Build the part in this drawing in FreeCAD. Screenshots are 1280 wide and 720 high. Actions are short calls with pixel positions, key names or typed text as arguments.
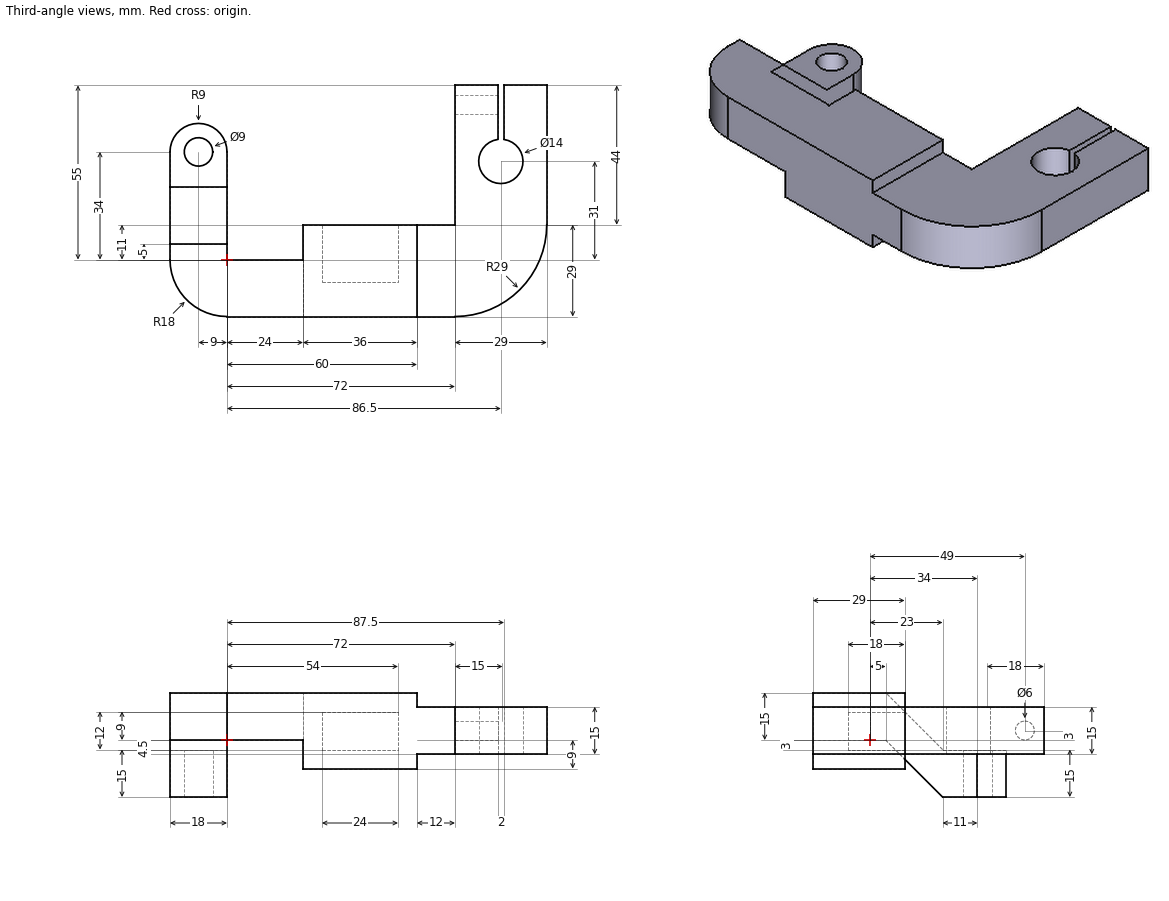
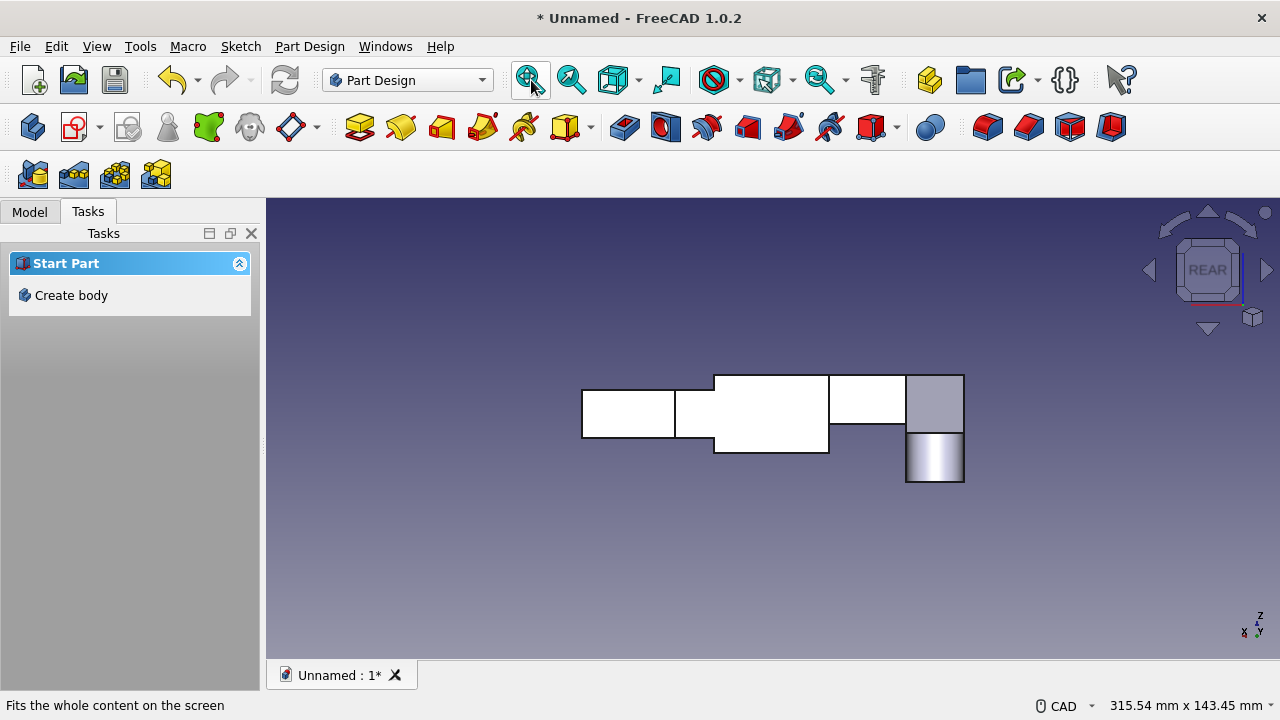
click(615, 413)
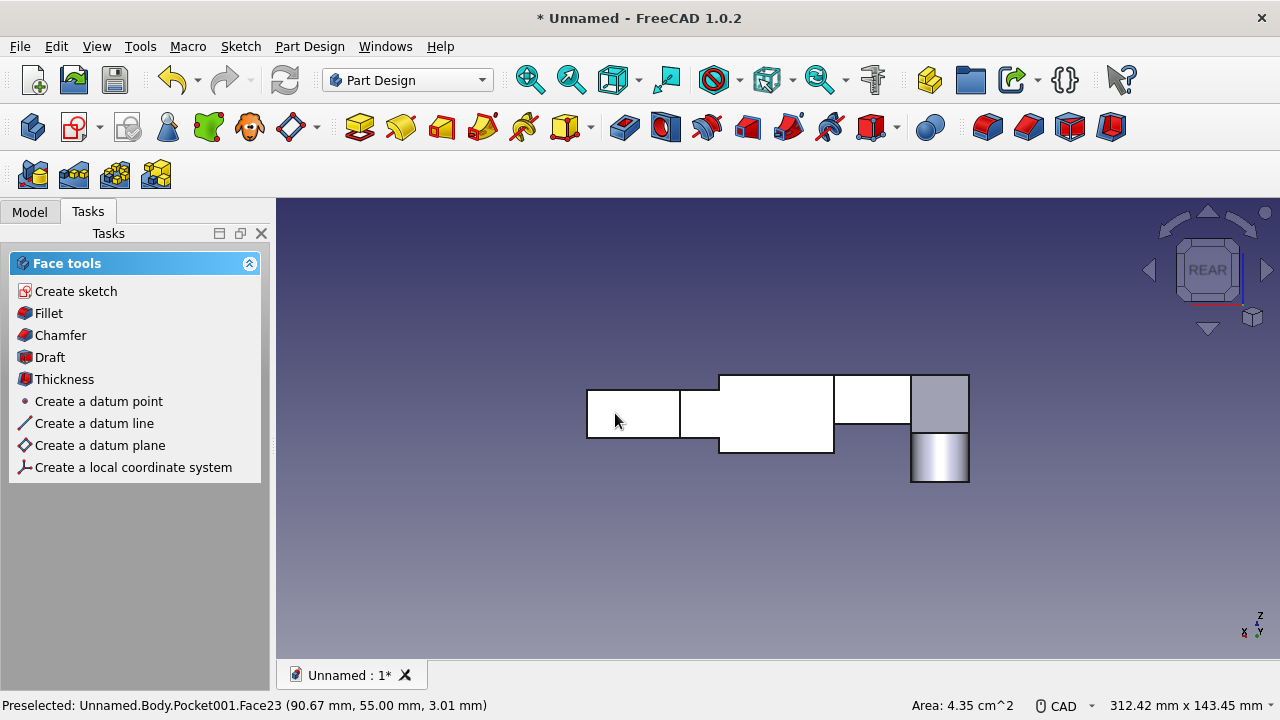
click(74, 128)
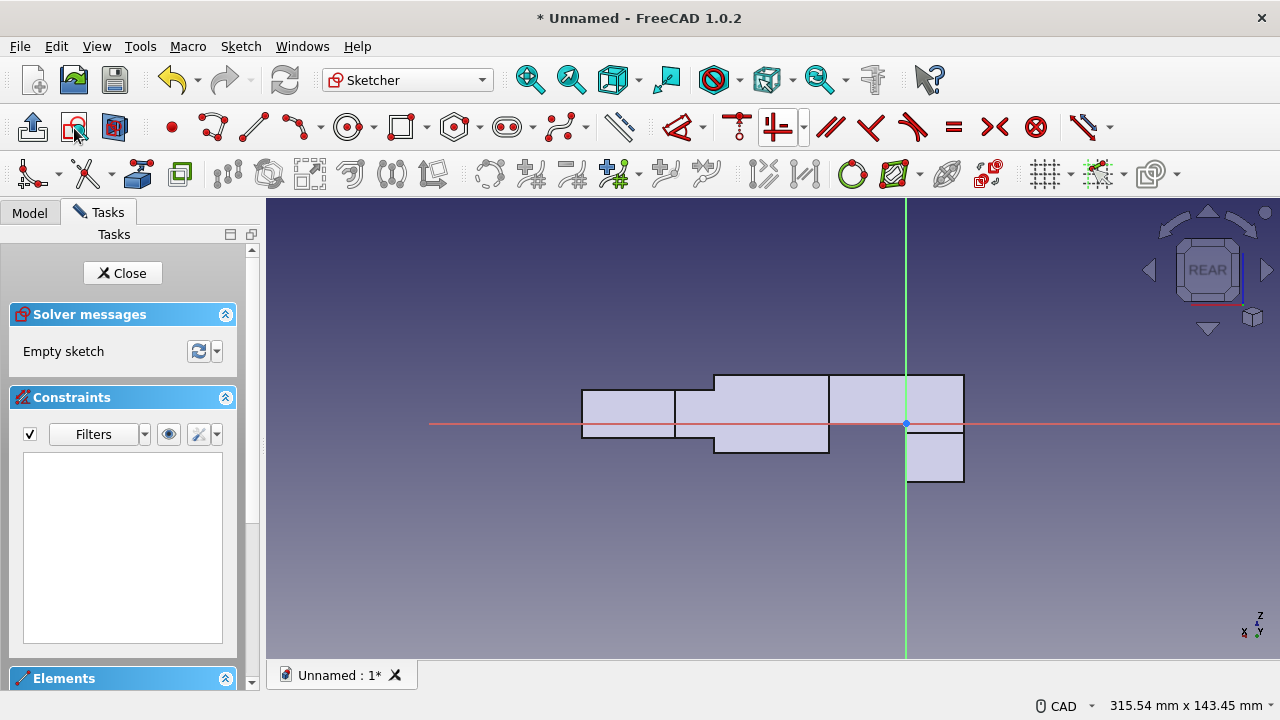
scroll(613, 411, up, 9)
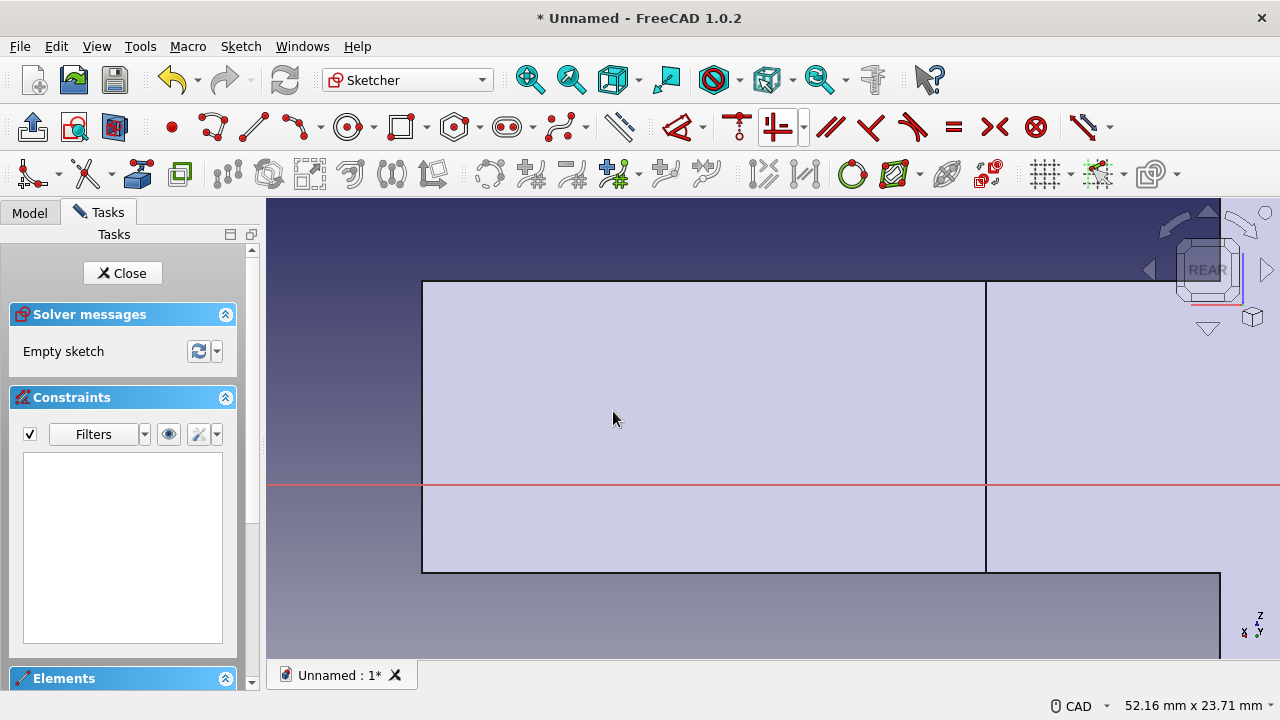
click(400, 128)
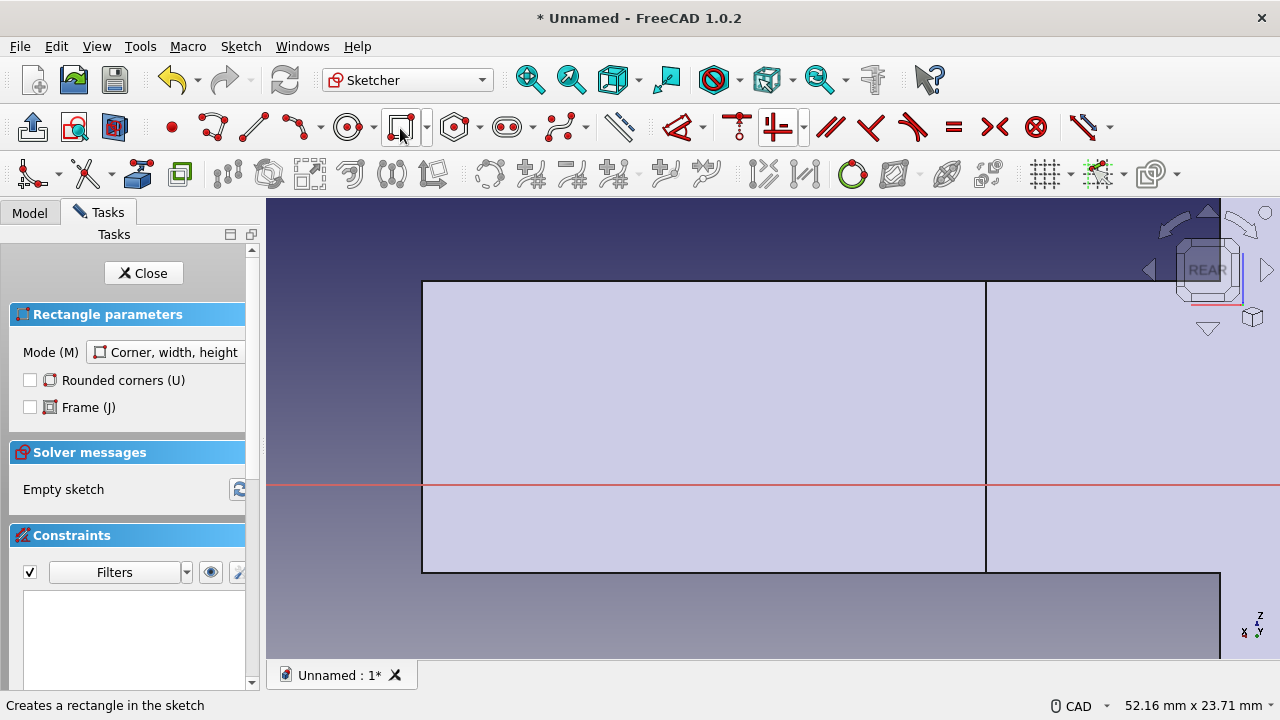
click(685, 281)
move(724, 573)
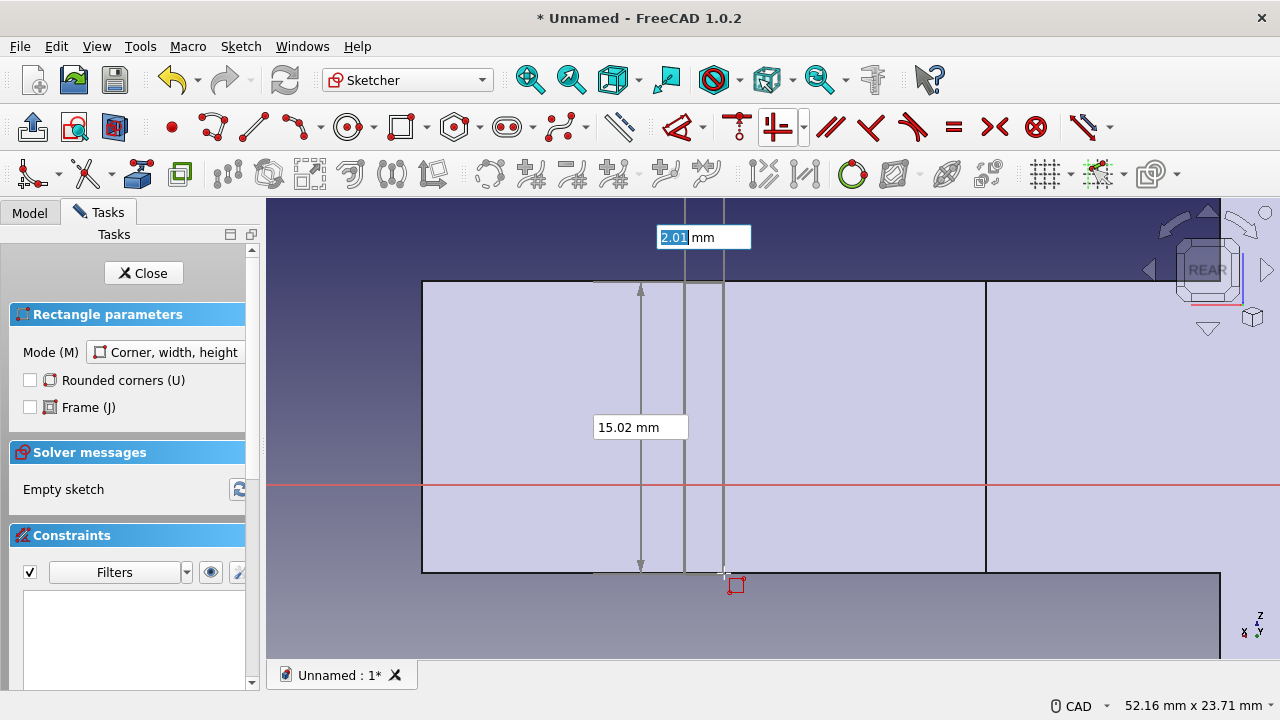
text(2)
key(Tab)
text(15)
key(Return)
key(Escape)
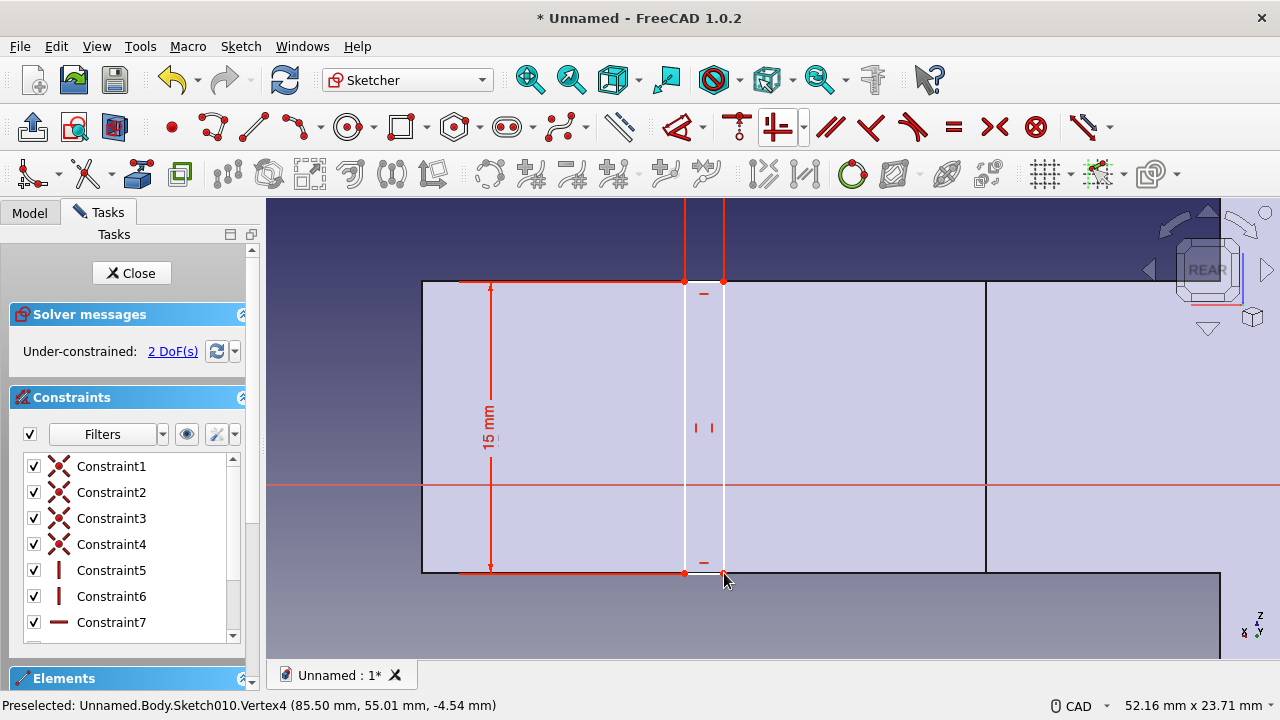
click(676, 128)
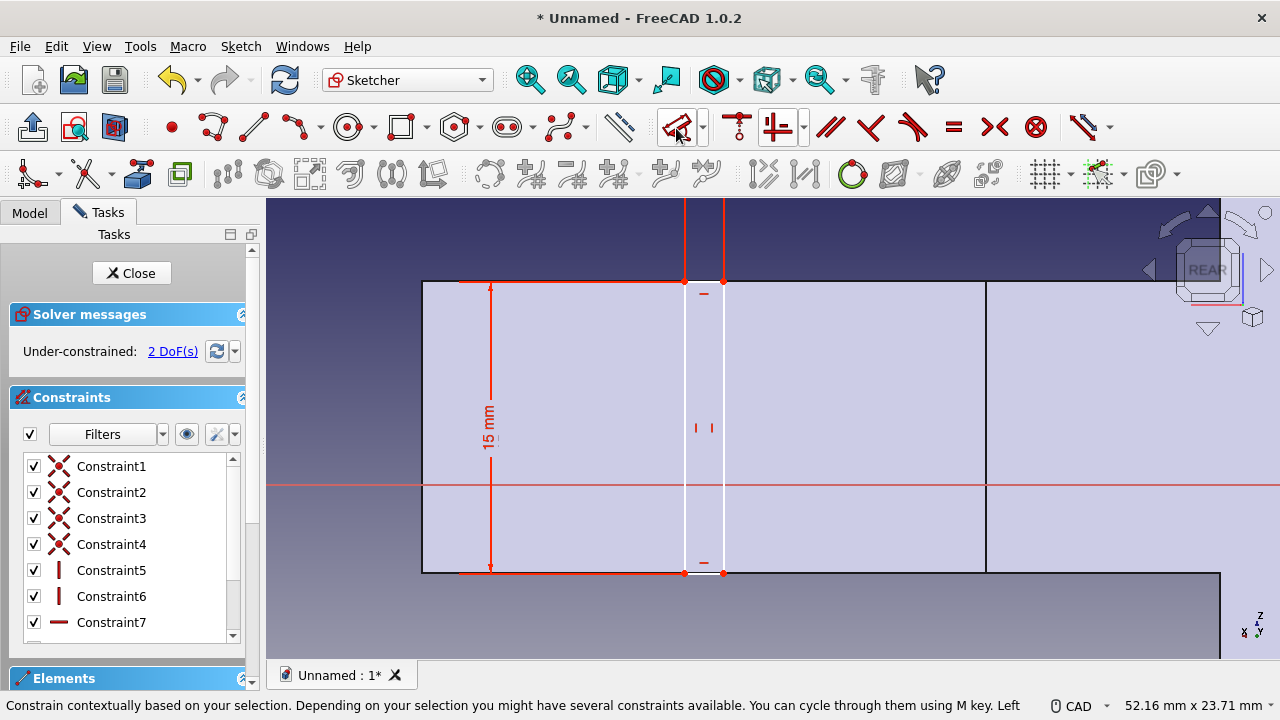
click(685, 574)
click(651, 529)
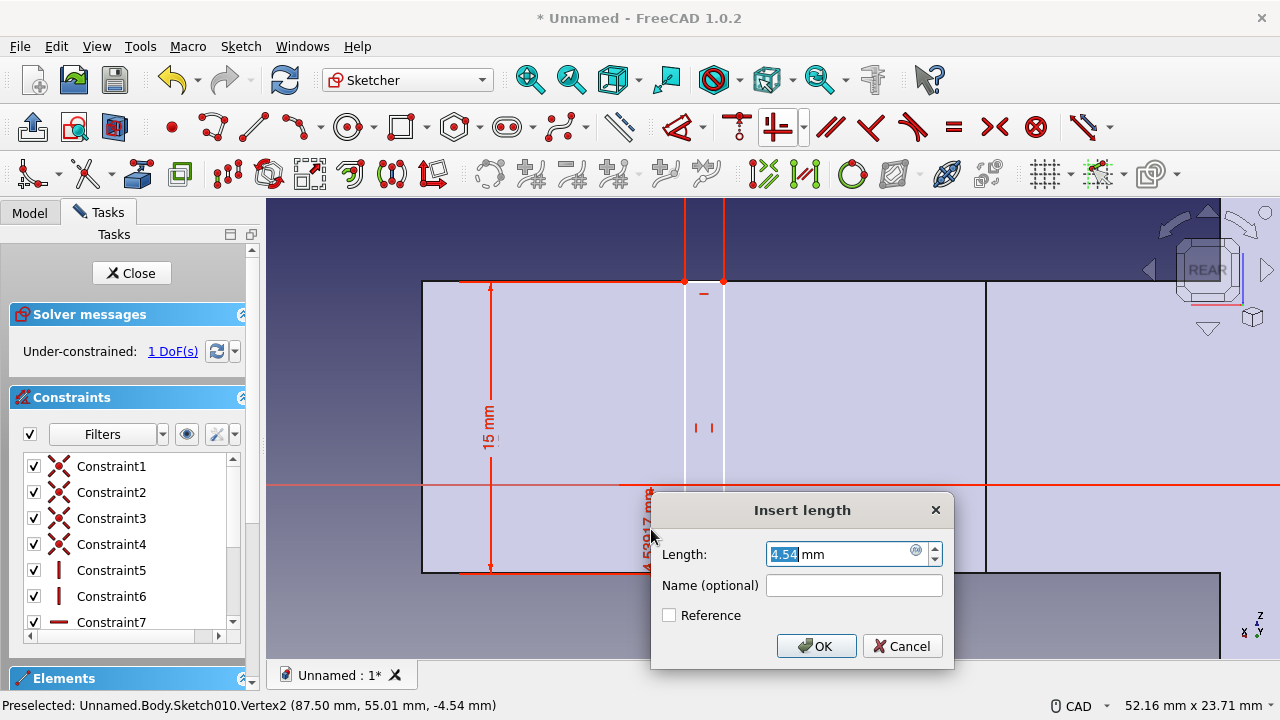
text(4.5)
key(Return)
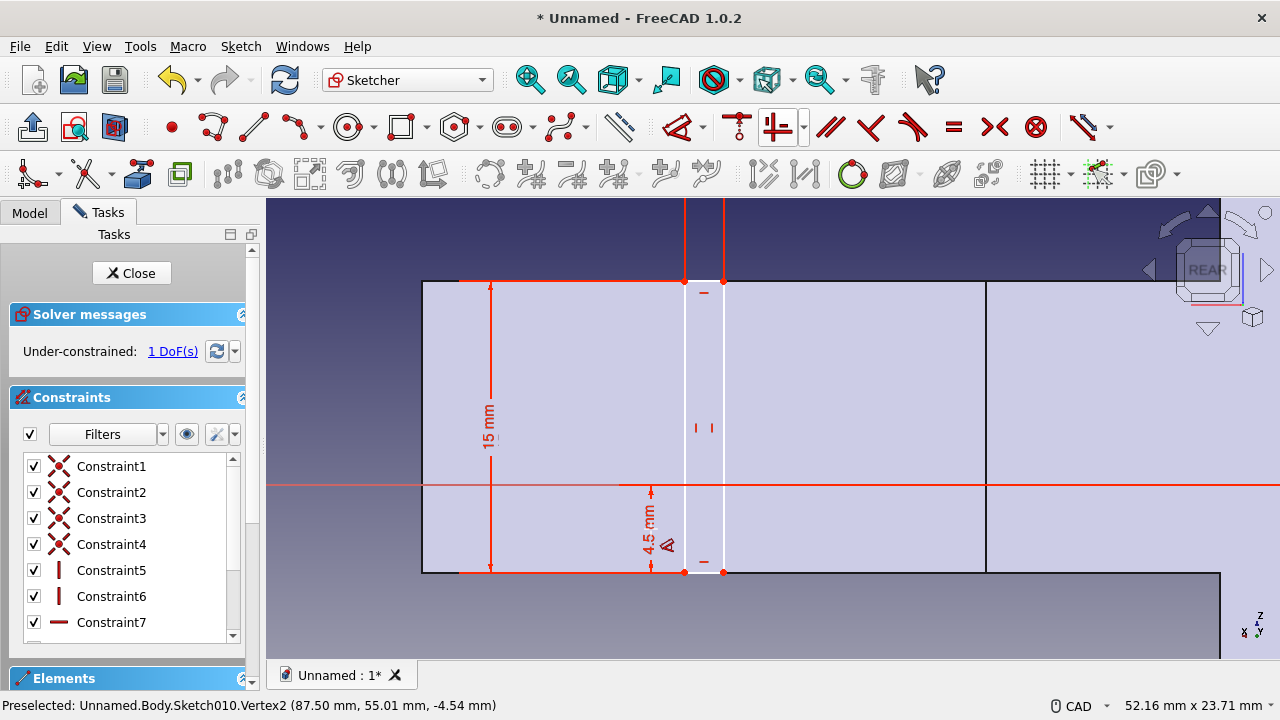
click(685, 281)
click(900, 247)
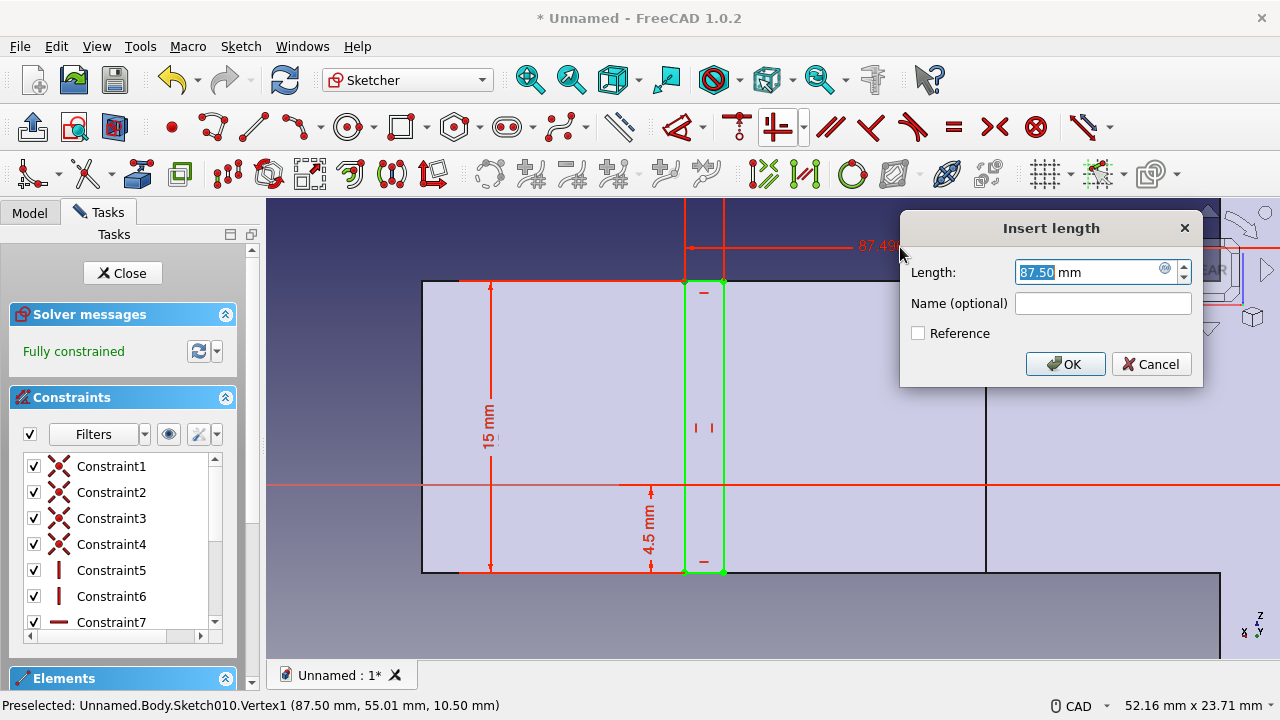
text(87.5)
key(Return)
key(Escape)